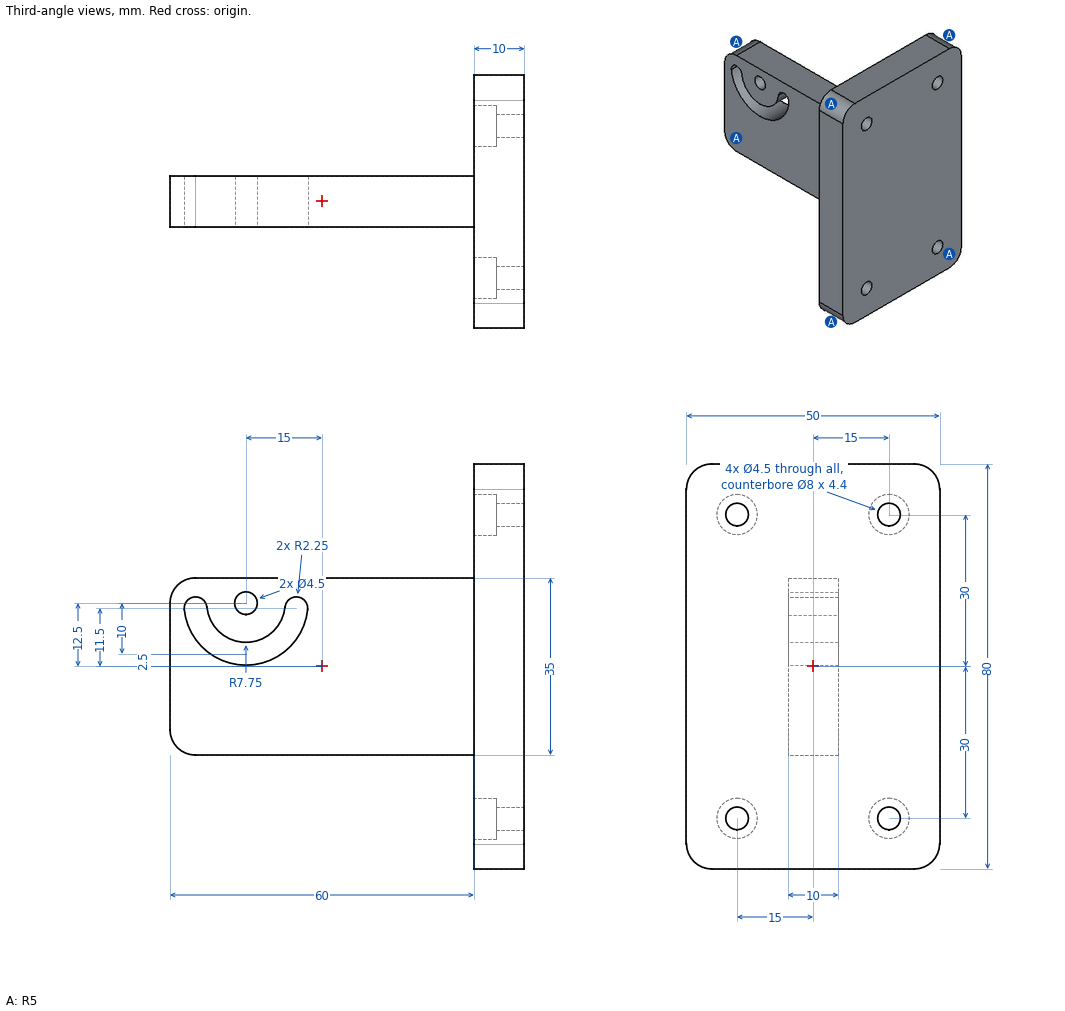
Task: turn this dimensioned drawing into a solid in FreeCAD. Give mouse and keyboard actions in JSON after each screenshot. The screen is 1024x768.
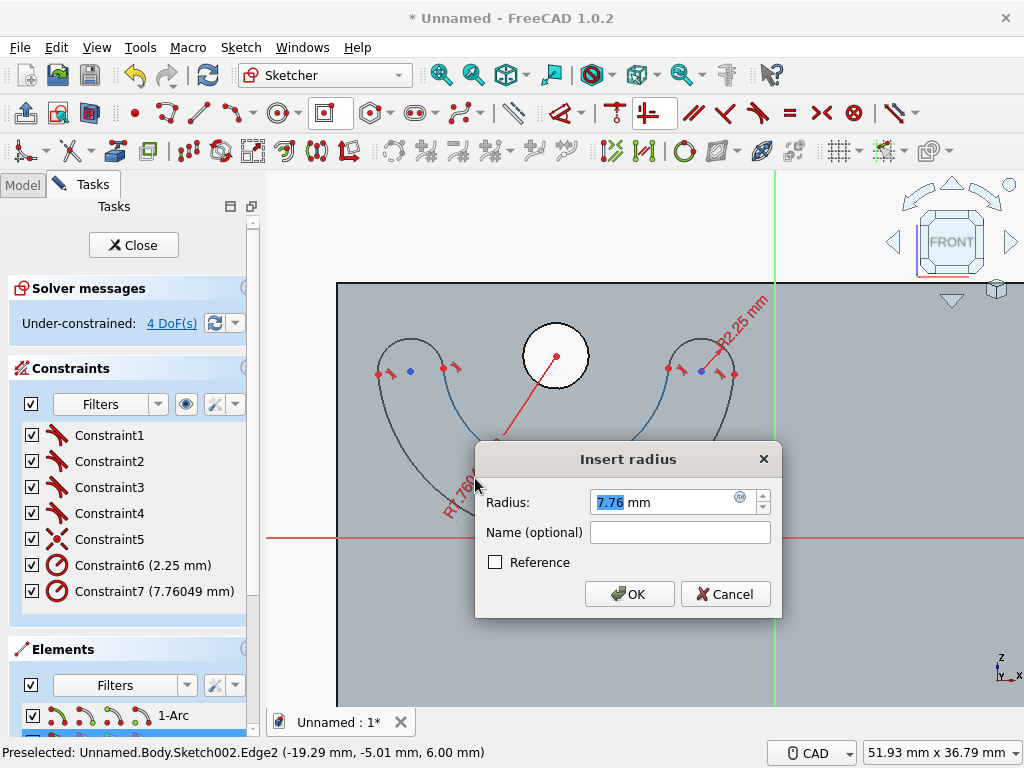
{"action": "type", "text": "7.75"}
{"action": "key", "text": "Return"}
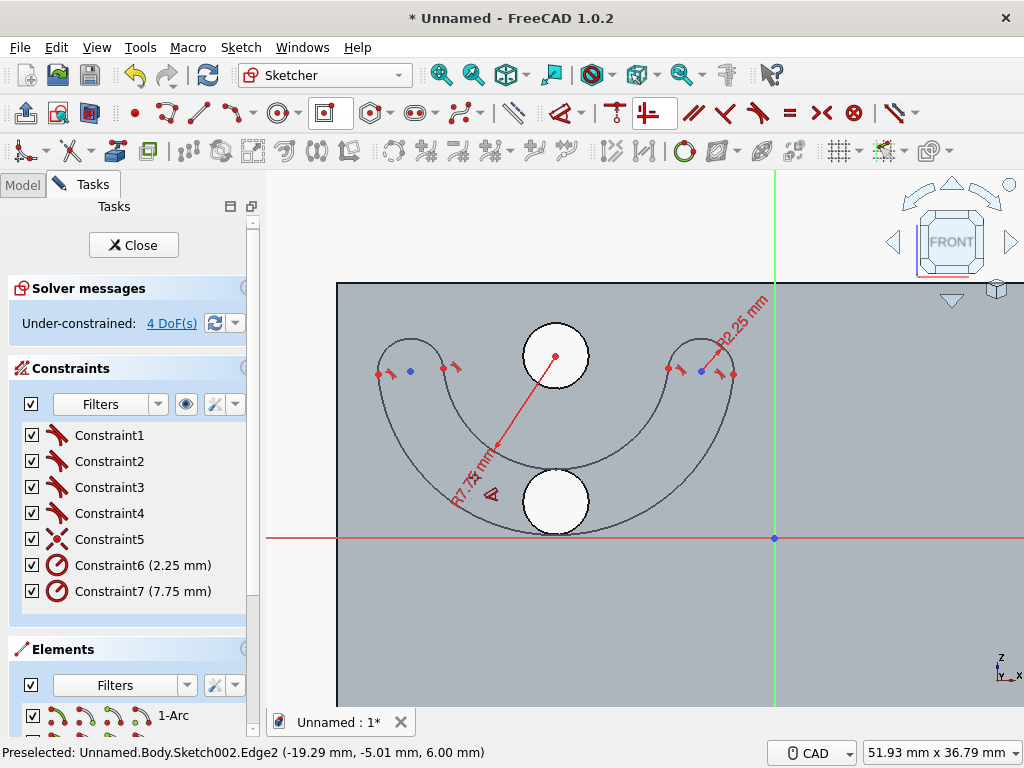
{"action": "left_click", "coordinate": [556, 356]}
{"action": "left_click", "coordinate": [665, 572]}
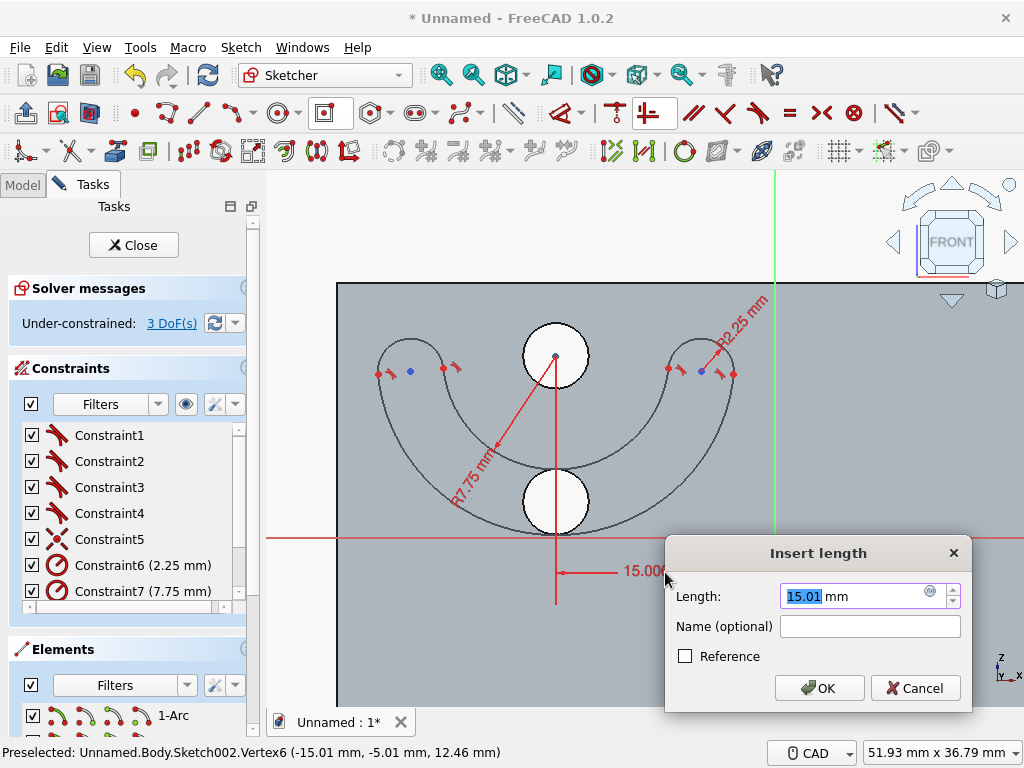
{"action": "type", "text": "15"}
{"action": "key", "text": "Return"}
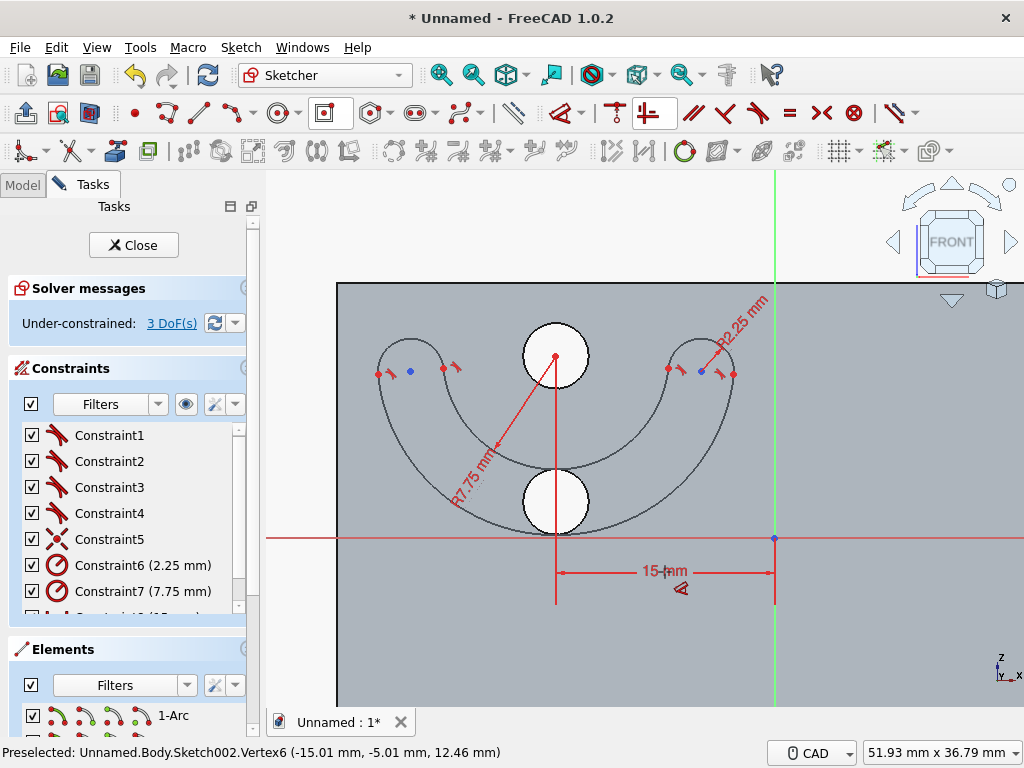
{"action": "left_click", "coordinate": [701, 372]}
{"action": "left_click", "coordinate": [809, 455]}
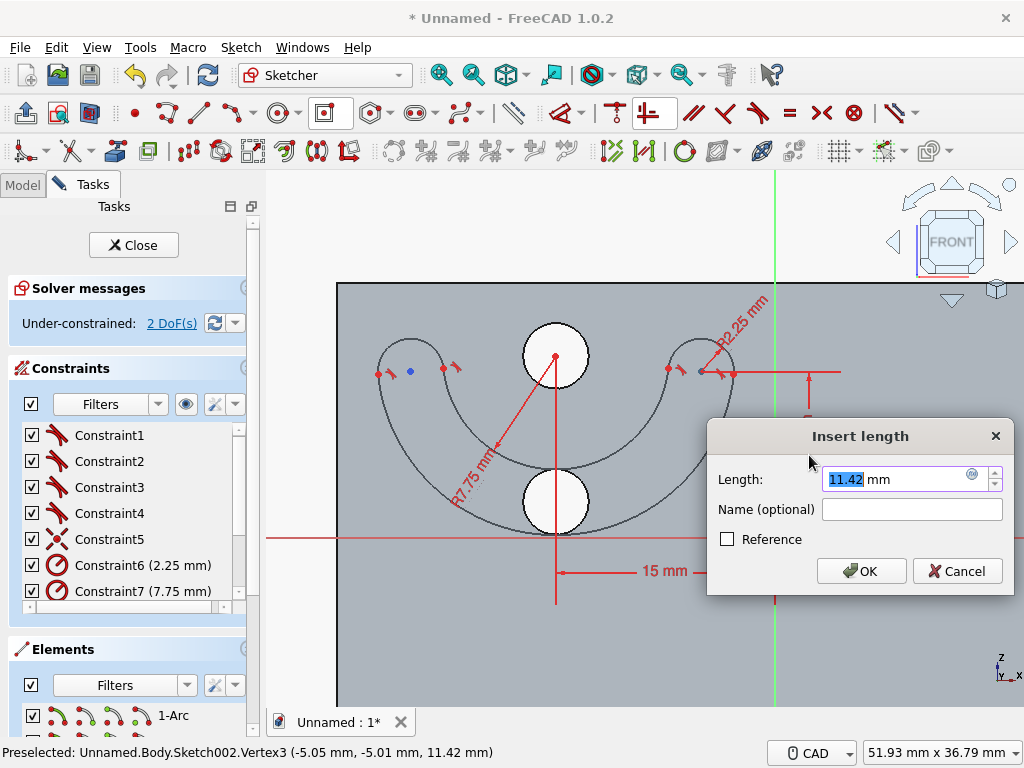
{"action": "type", "text": "11.5"}
{"action": "key", "text": "Return"}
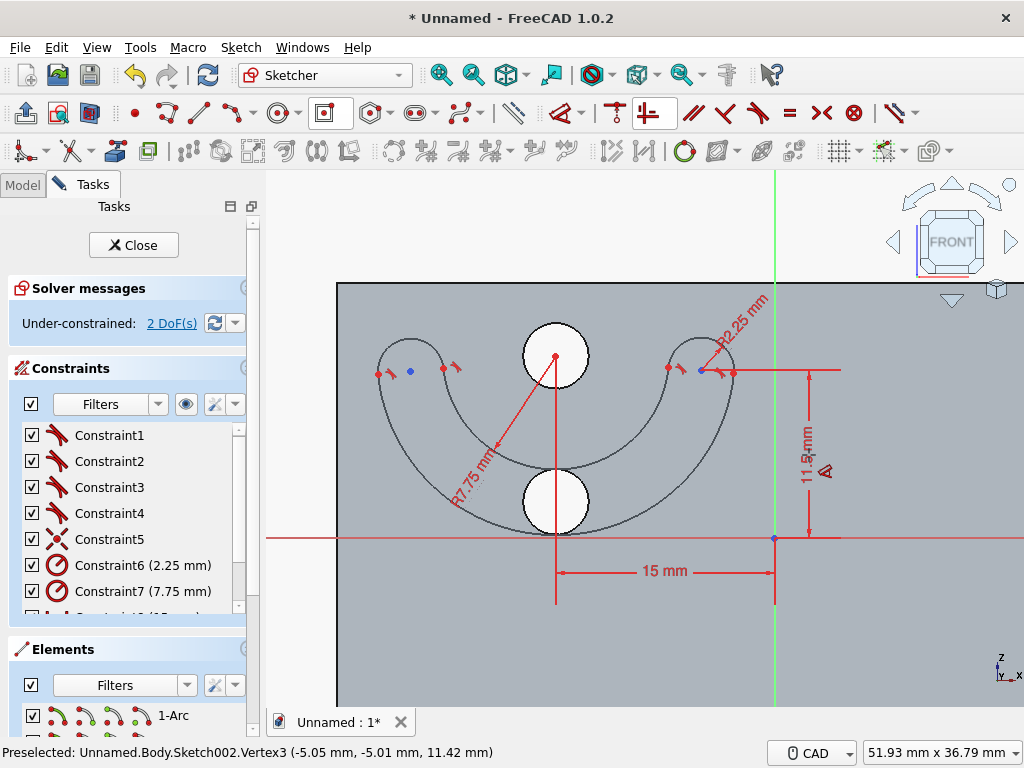
{"action": "left_click", "coordinate": [556, 356]}
{"action": "left_click", "coordinate": [809, 406]}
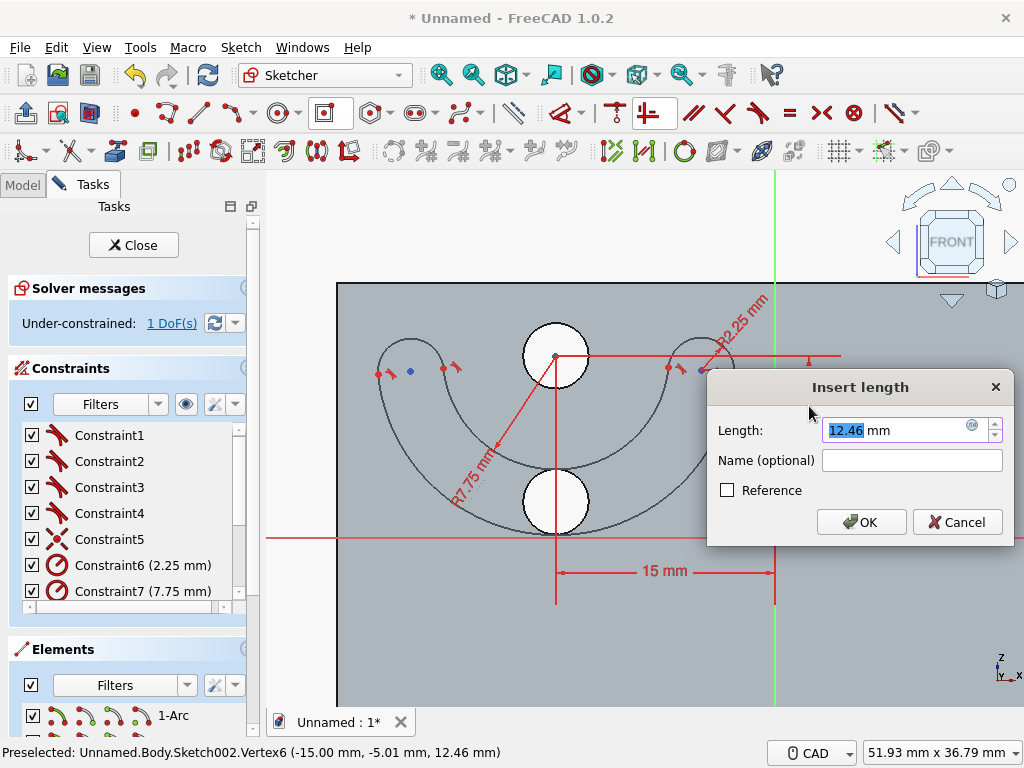
{"action": "type", "text": "12.5"}
{"action": "key", "text": "Return"}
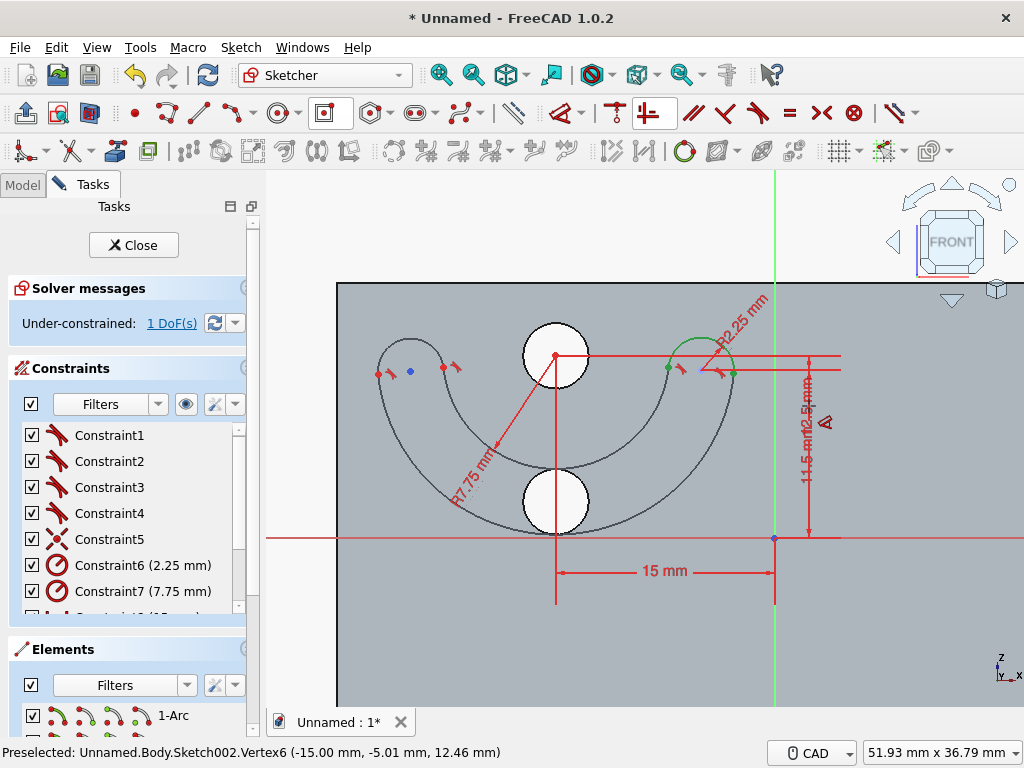
{"action": "left_click", "coordinate": [411, 371]}
{"action": "left_click", "coordinate": [809, 493]}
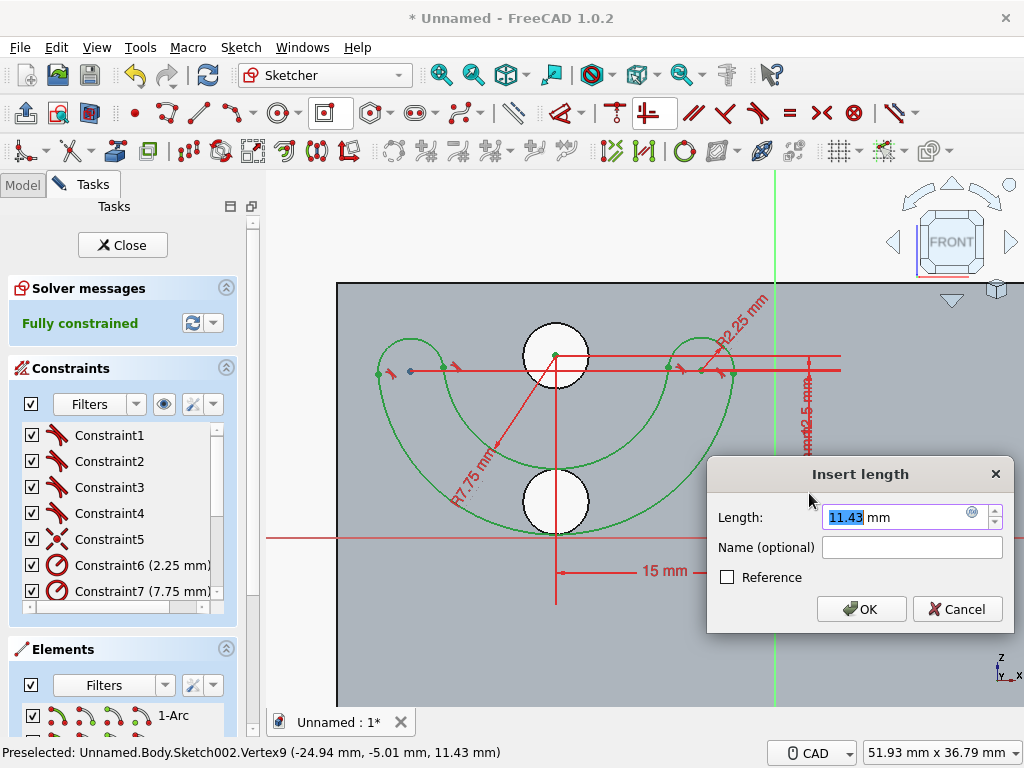
{"action": "type", "text": "11.5"}
{"action": "key", "text": "Return"}
{"action": "key", "text": "Escape"}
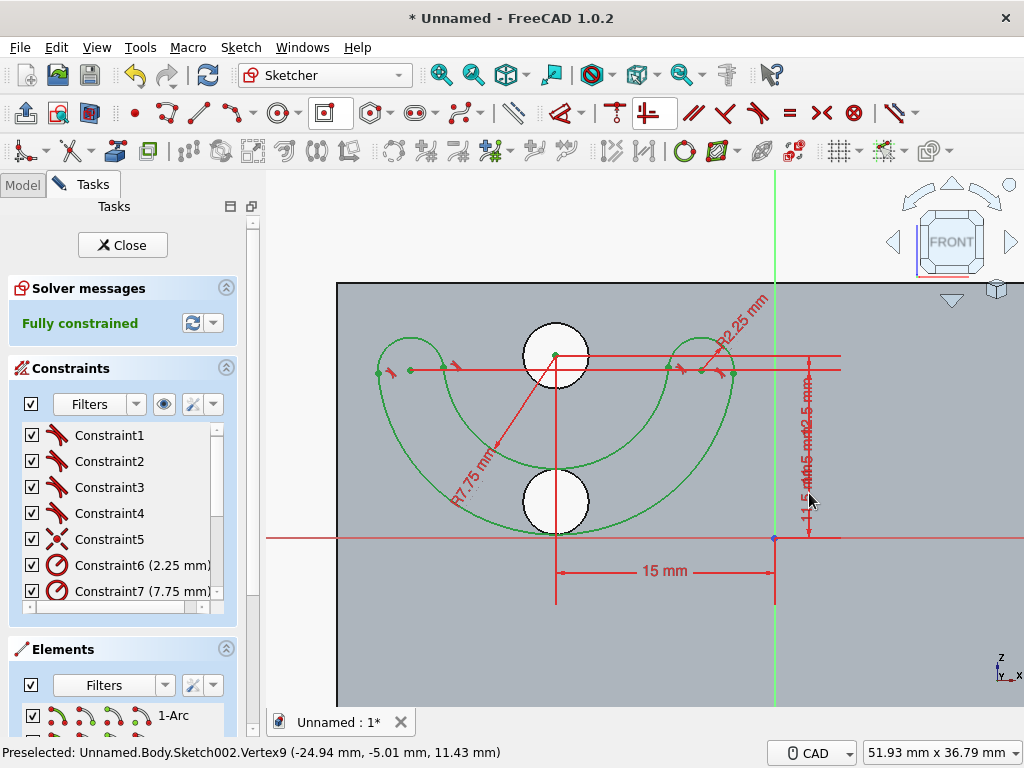
{"action": "left_click", "coordinate": [123, 245]}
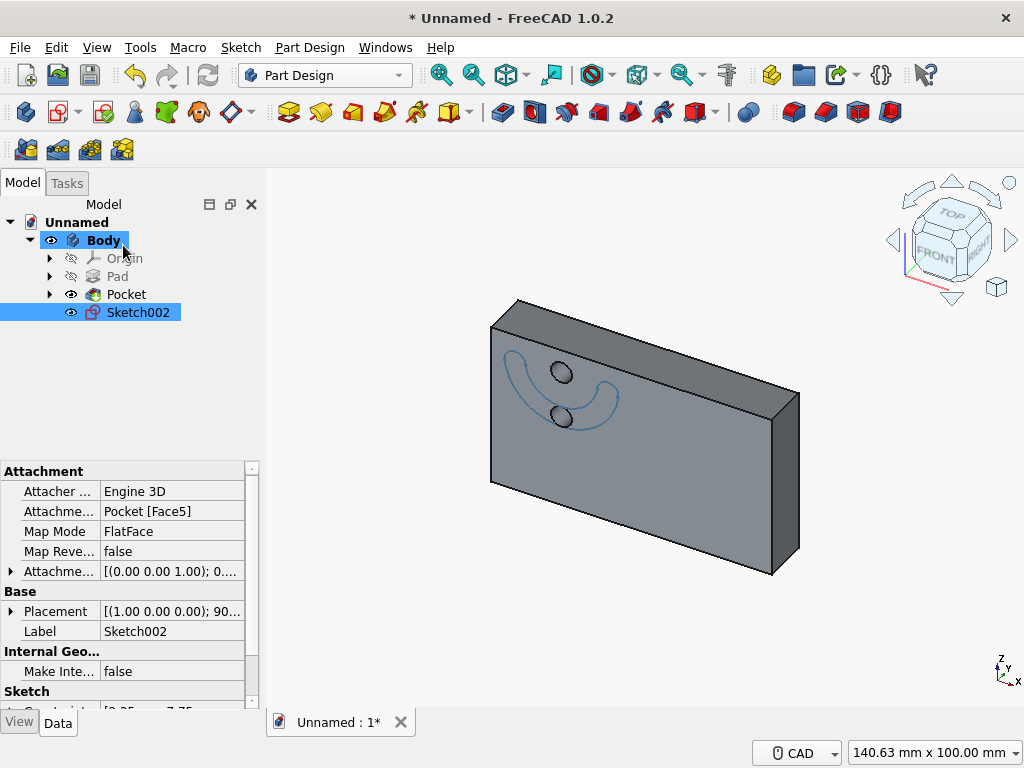
{"action": "left_click", "coordinate": [504, 112]}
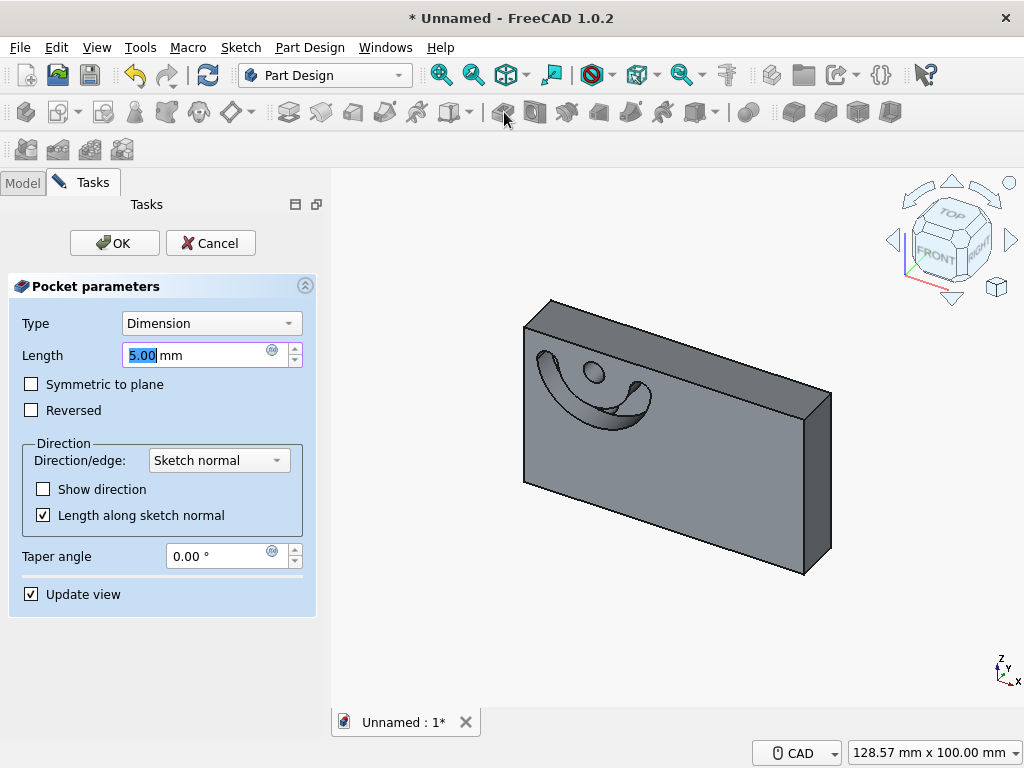
{"action": "left_click", "coordinate": [212, 324]}